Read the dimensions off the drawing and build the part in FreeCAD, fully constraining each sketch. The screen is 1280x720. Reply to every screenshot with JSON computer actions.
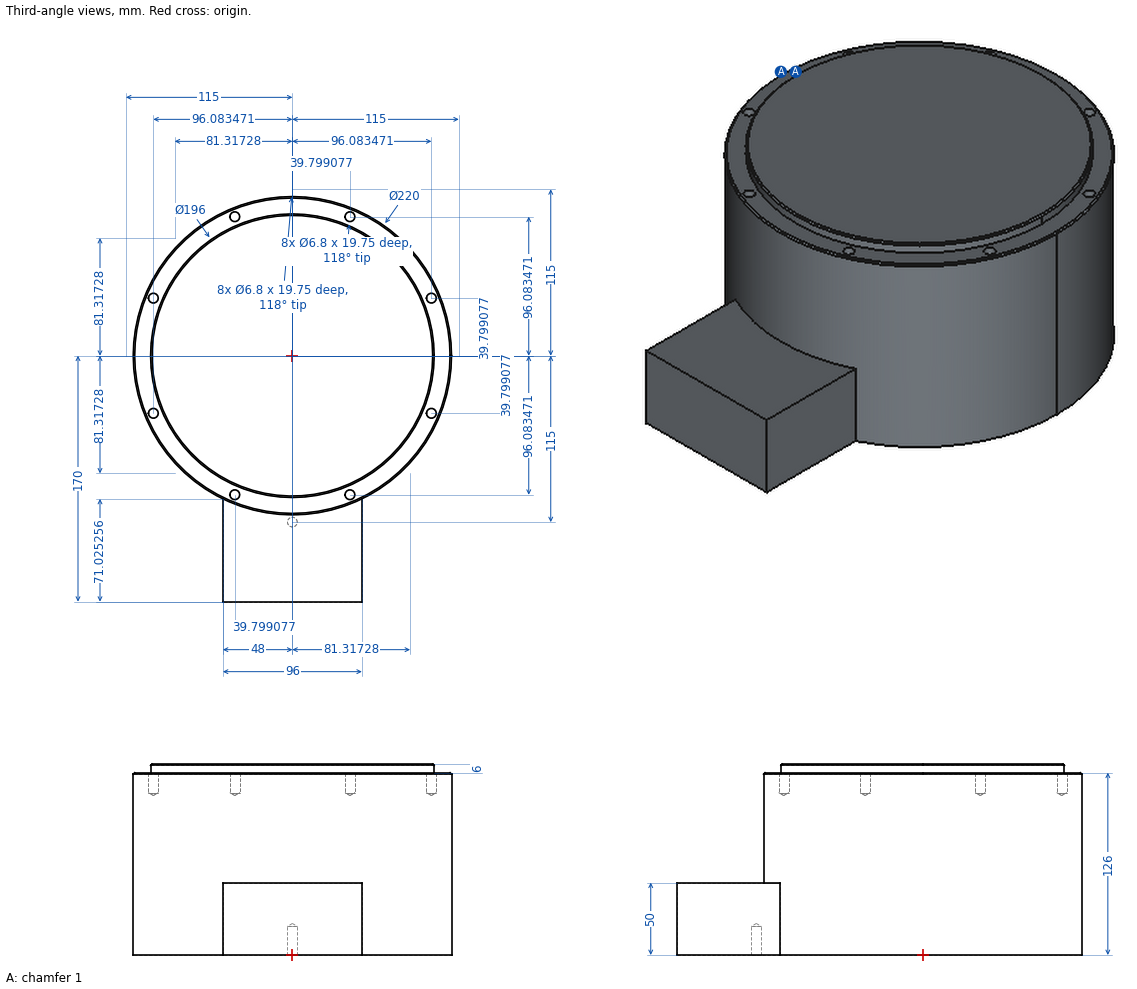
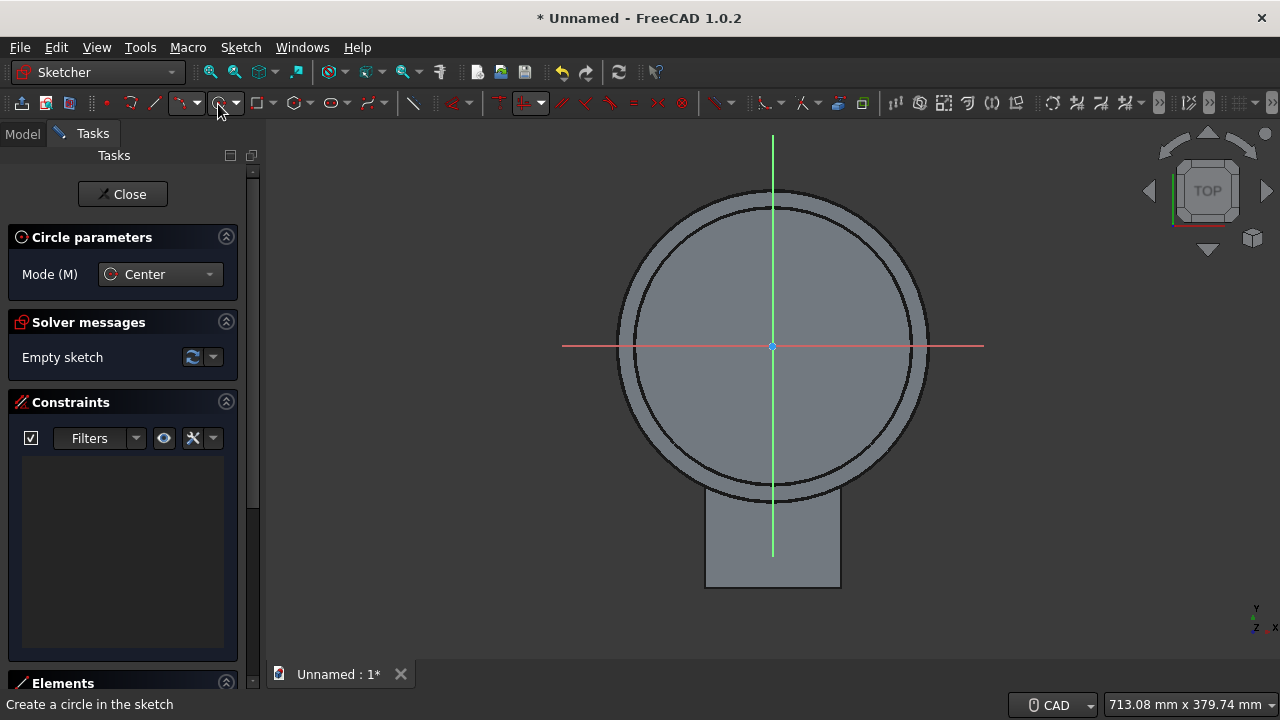
{"action": "scroll", "coordinate": [830, 210], "scroll_direction": "up", "scroll_amount": 8}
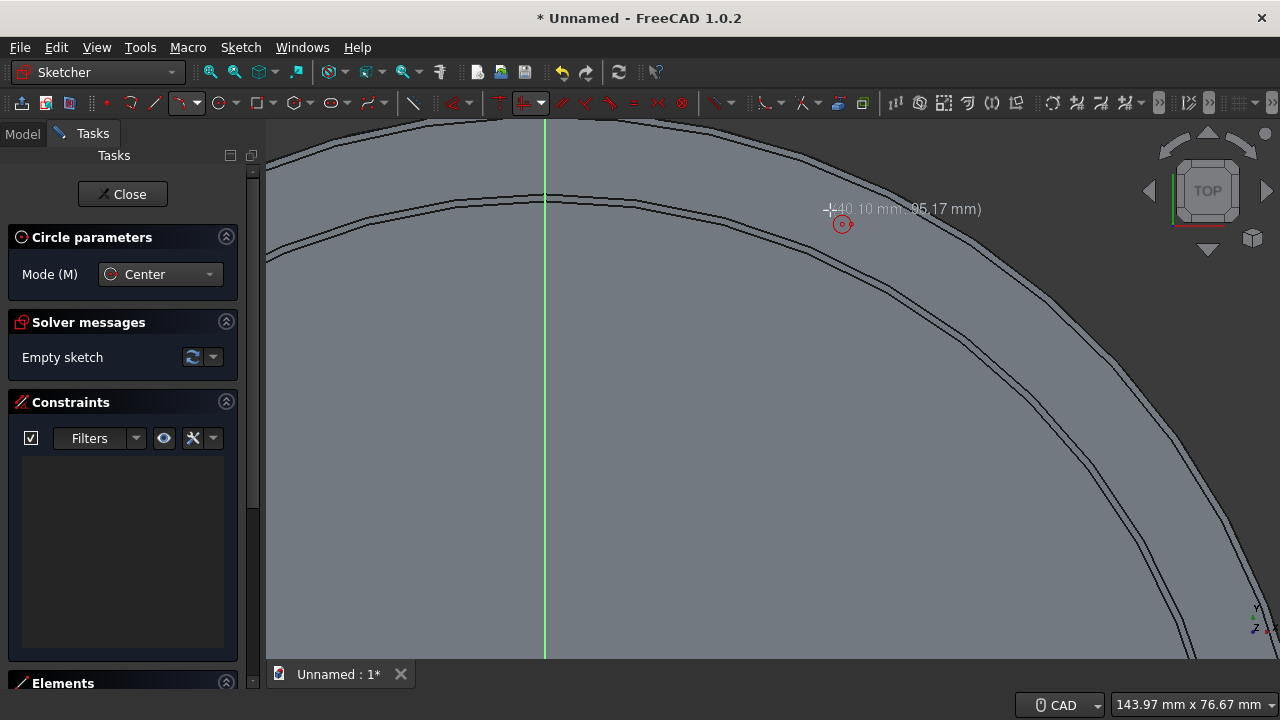
{"action": "scroll", "coordinate": [757, 227], "scroll_direction": "down", "scroll_amount": 7}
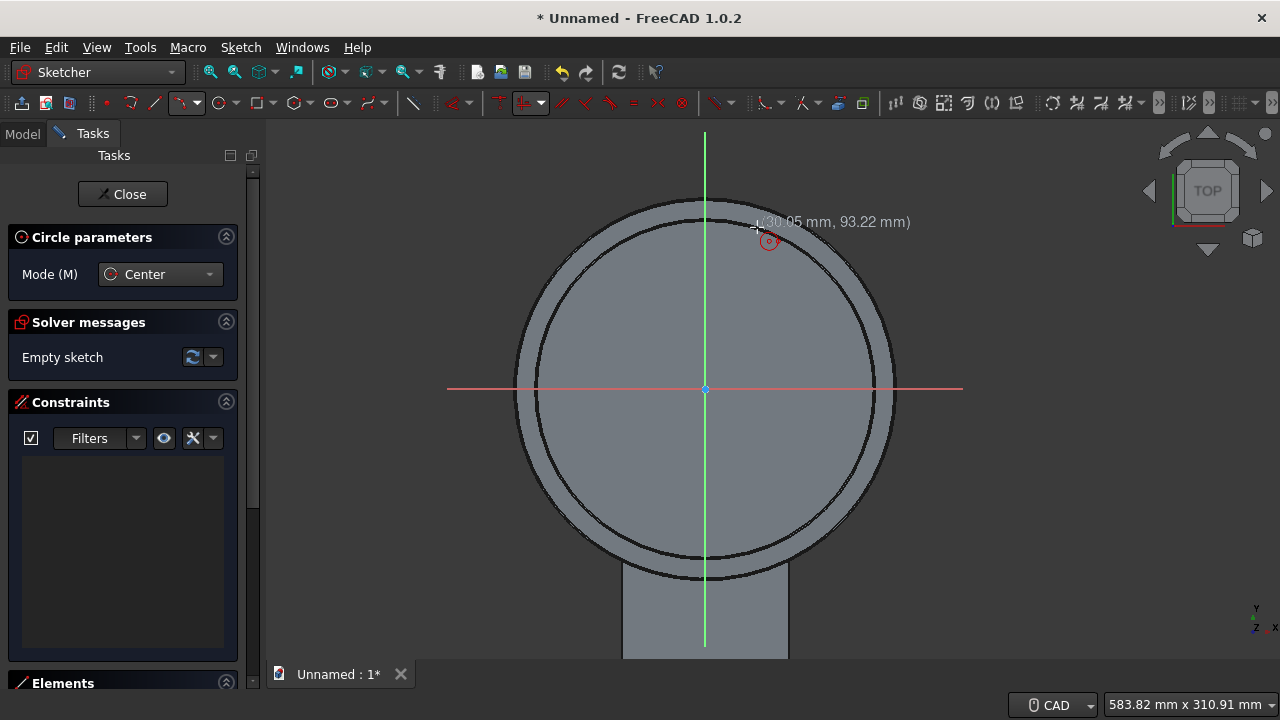
{"action": "left_click", "coordinate": [774, 222]}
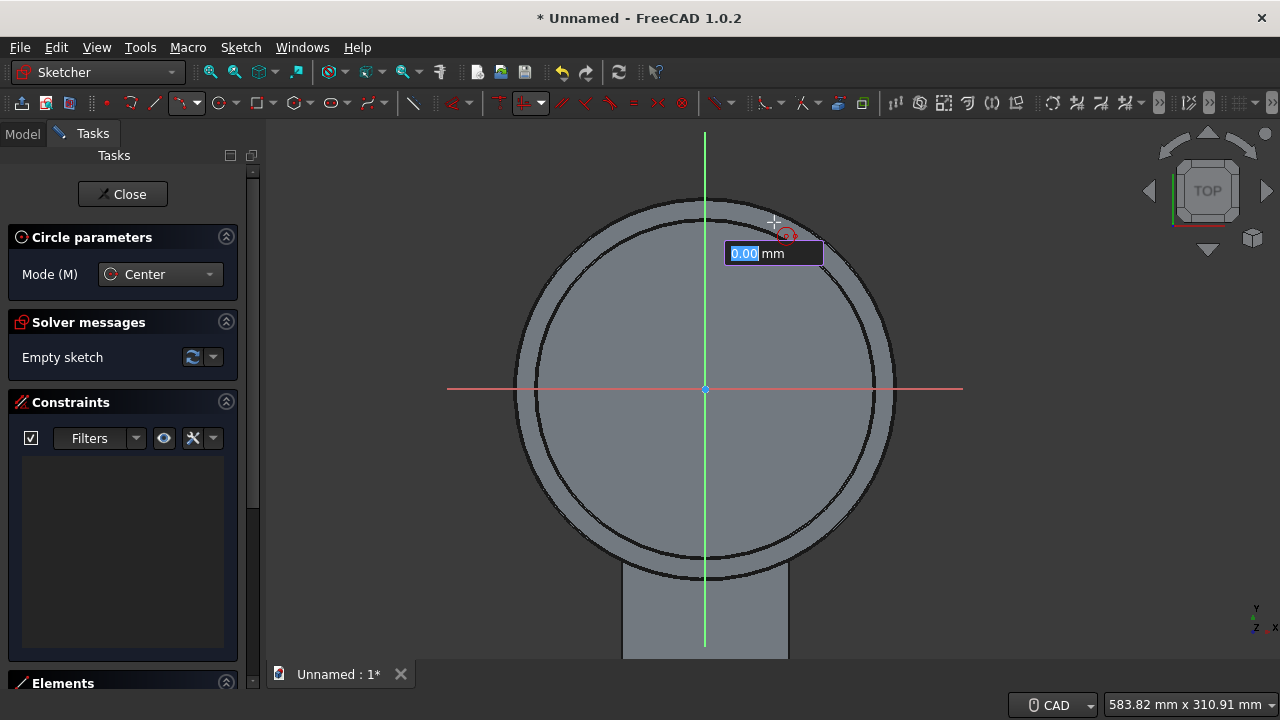
{"action": "scroll", "coordinate": [778, 218], "scroll_direction": "up", "scroll_amount": 5}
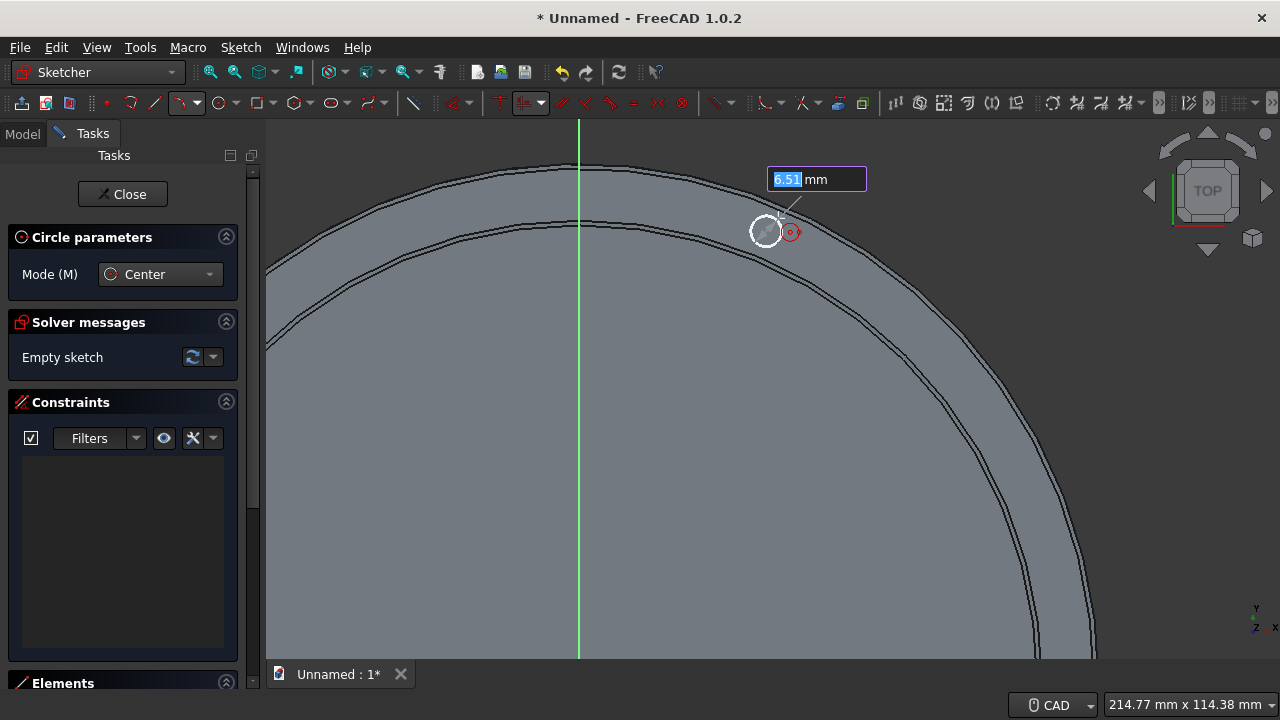
{"action": "left_click", "coordinate": [778, 218]}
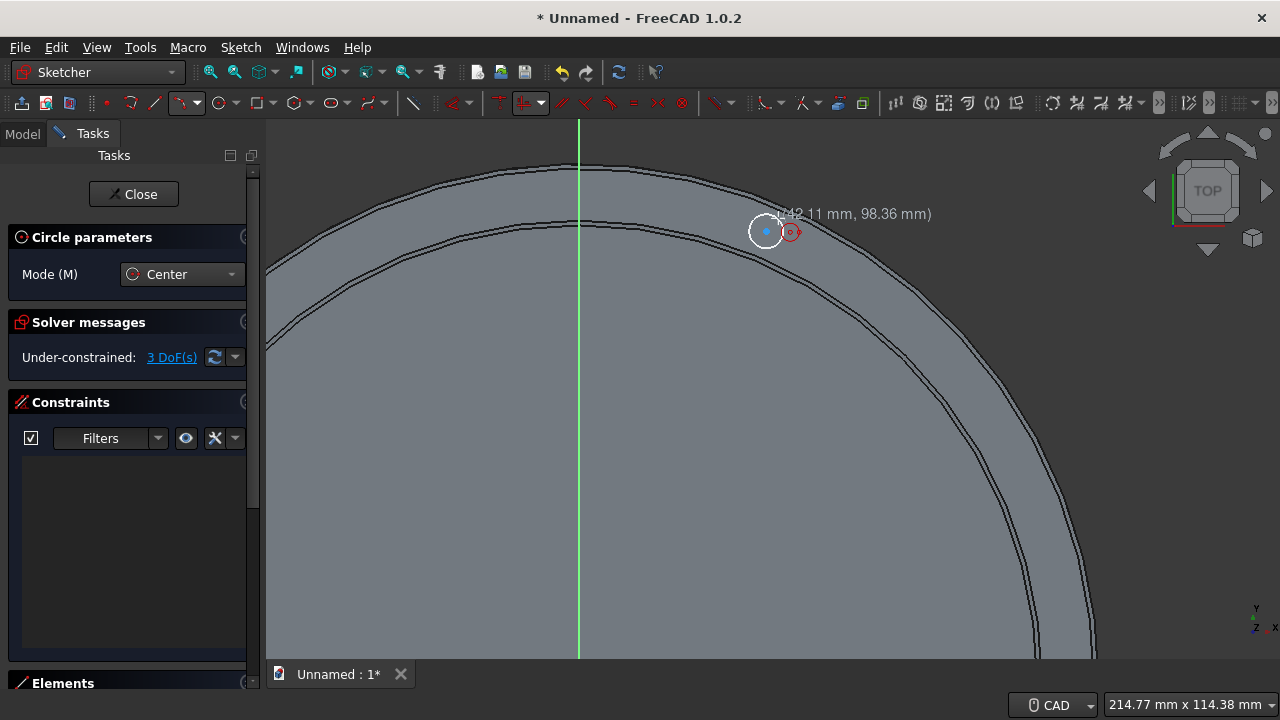
{"action": "scroll", "coordinate": [1033, 495], "scroll_direction": "up", "scroll_amount": 2}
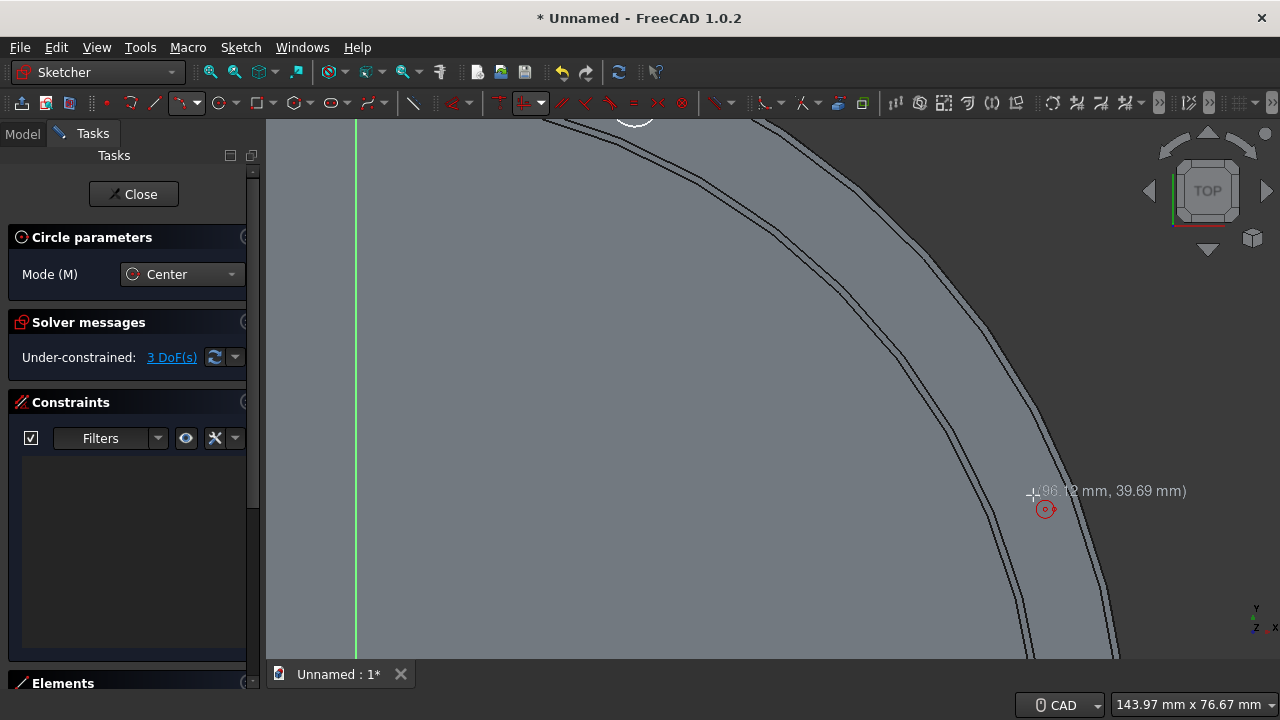
{"action": "scroll", "coordinate": [819, 262], "scroll_direction": "down", "scroll_amount": 7}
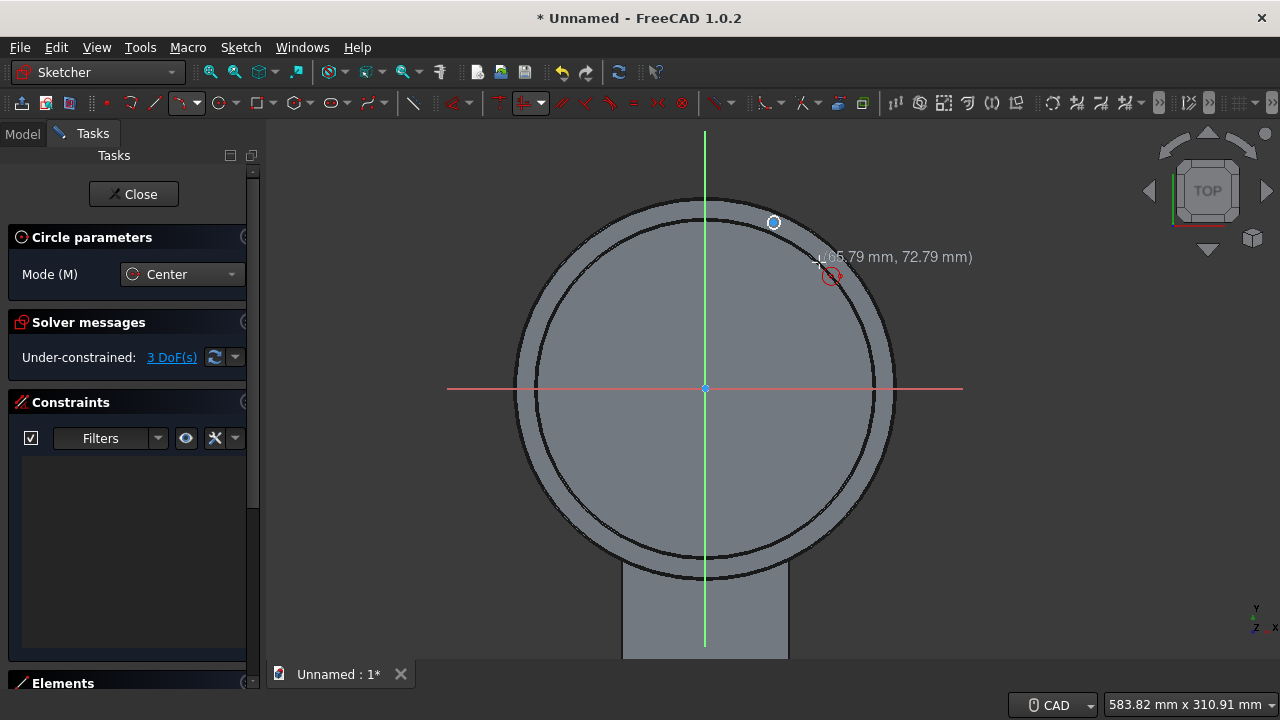
{"action": "left_click", "coordinate": [872, 320]}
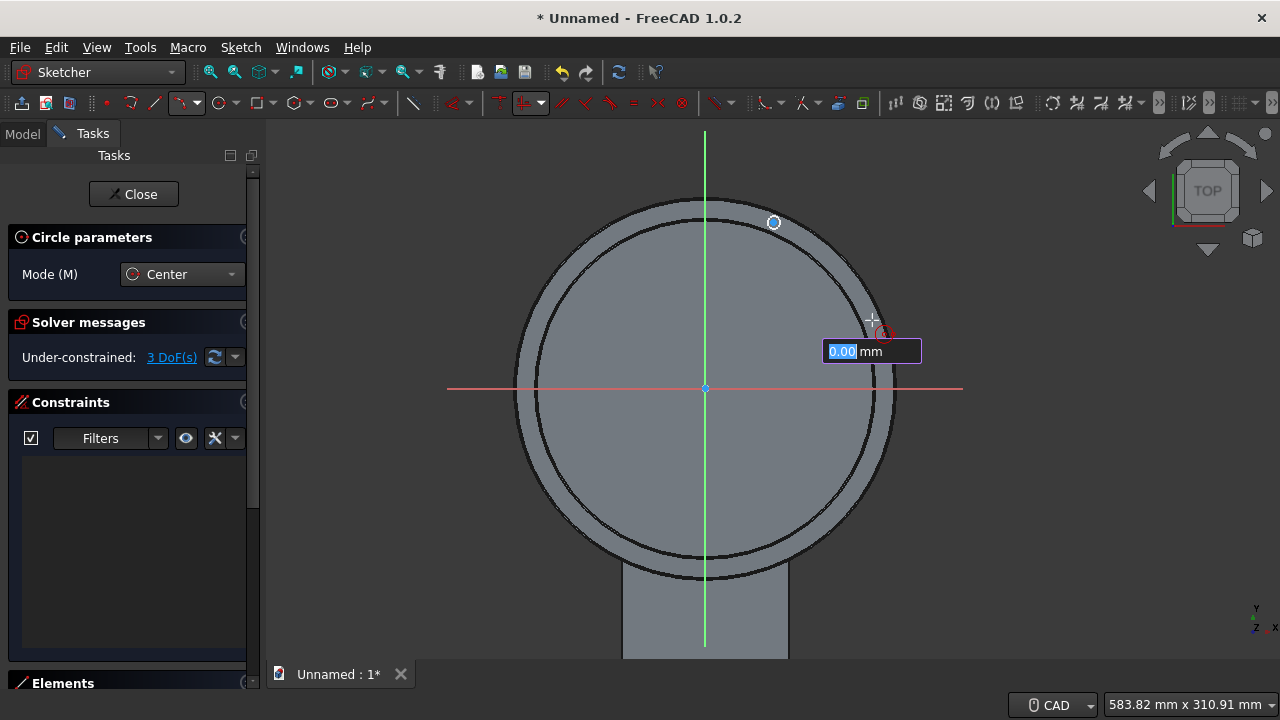
{"action": "scroll", "coordinate": [876, 316], "scroll_direction": "up", "scroll_amount": 5}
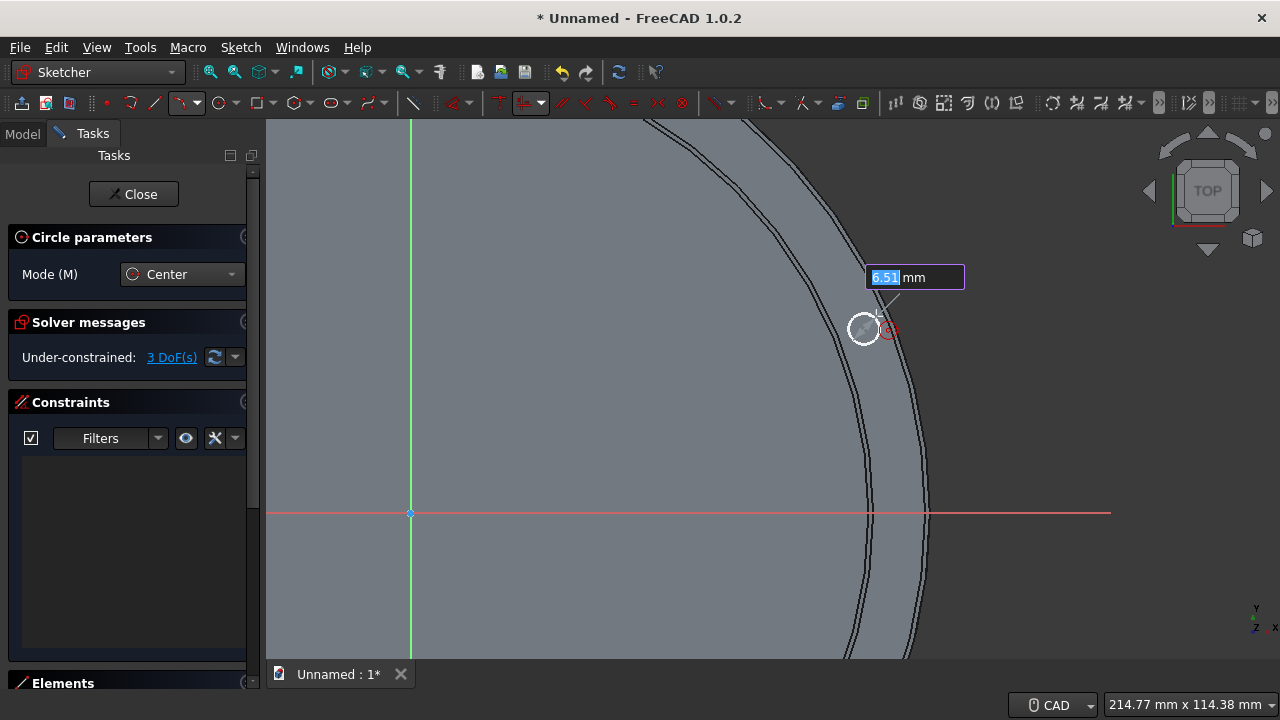
{"action": "left_click", "coordinate": [876, 314]}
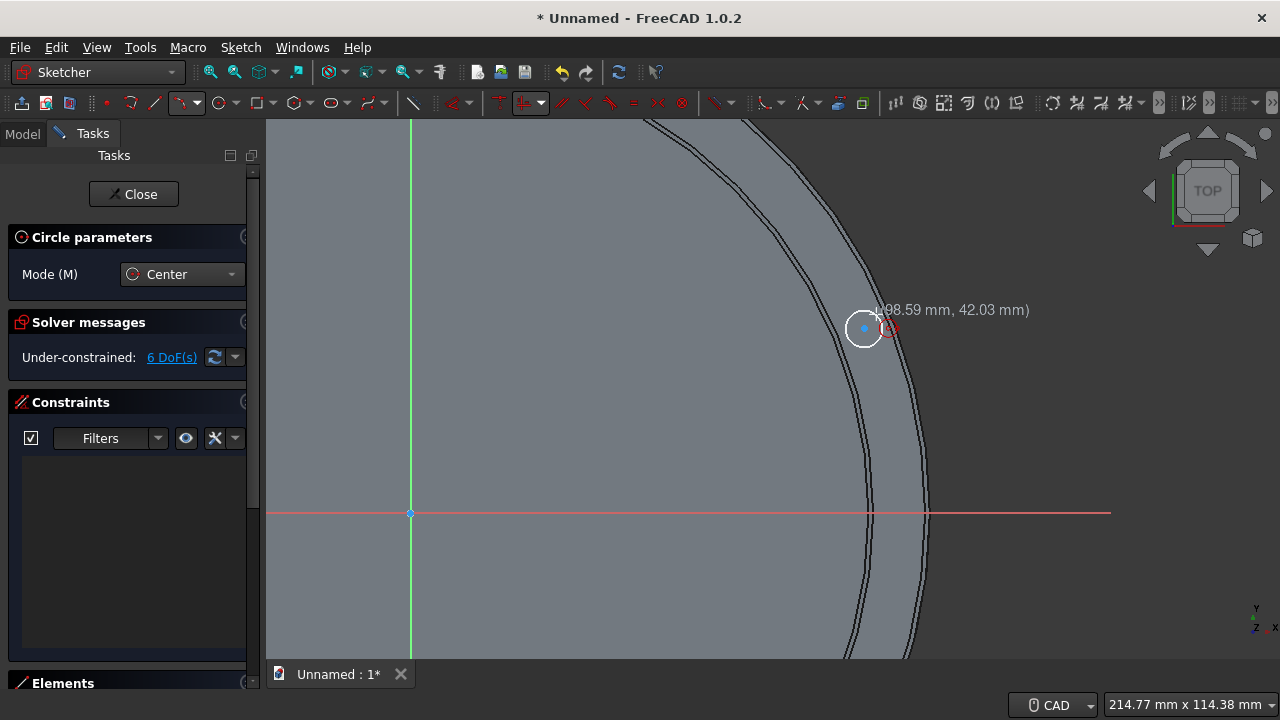
{"action": "scroll", "coordinate": [876, 317], "scroll_direction": "down", "scroll_amount": 5}